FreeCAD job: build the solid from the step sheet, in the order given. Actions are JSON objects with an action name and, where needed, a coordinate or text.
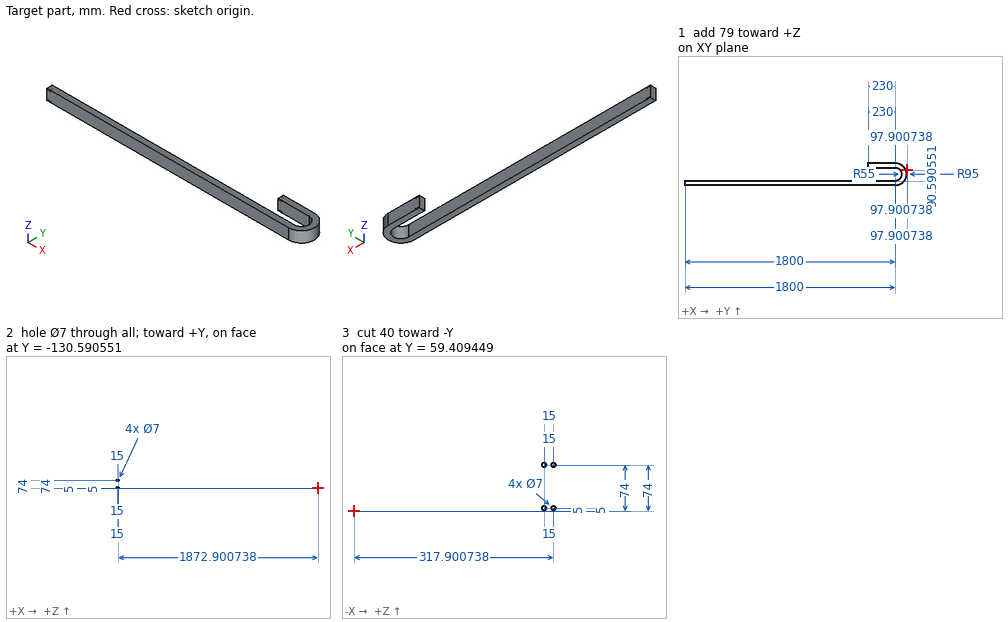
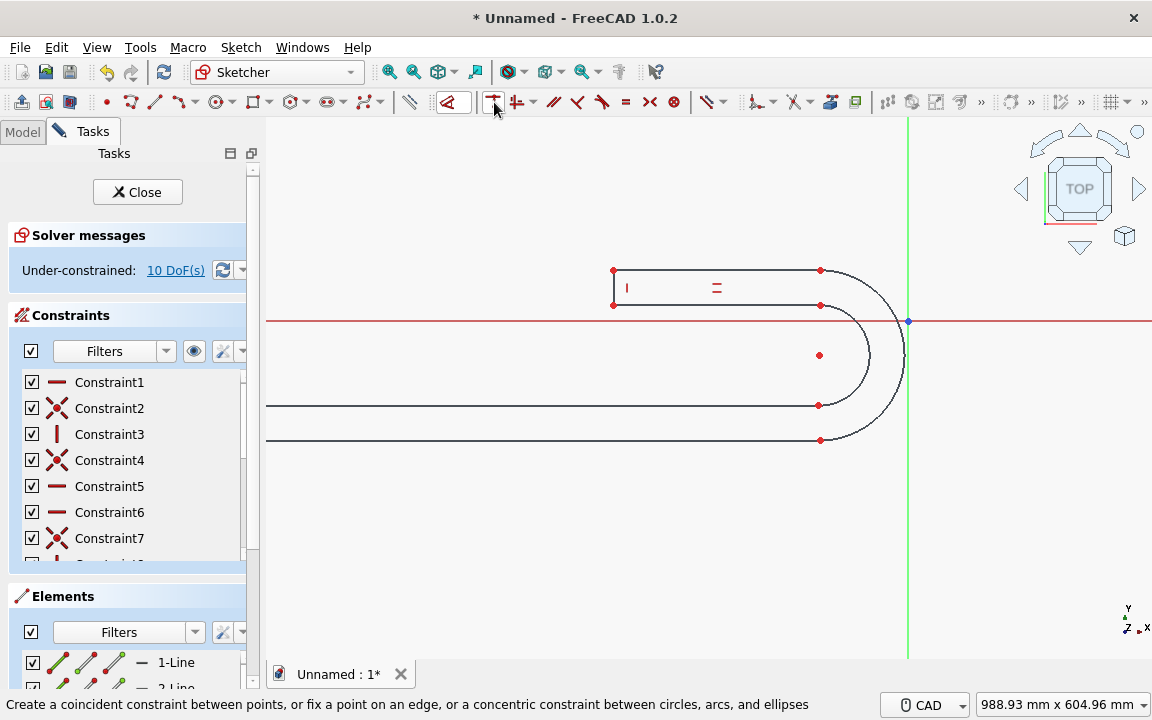
{"action": "key", "text": "d"}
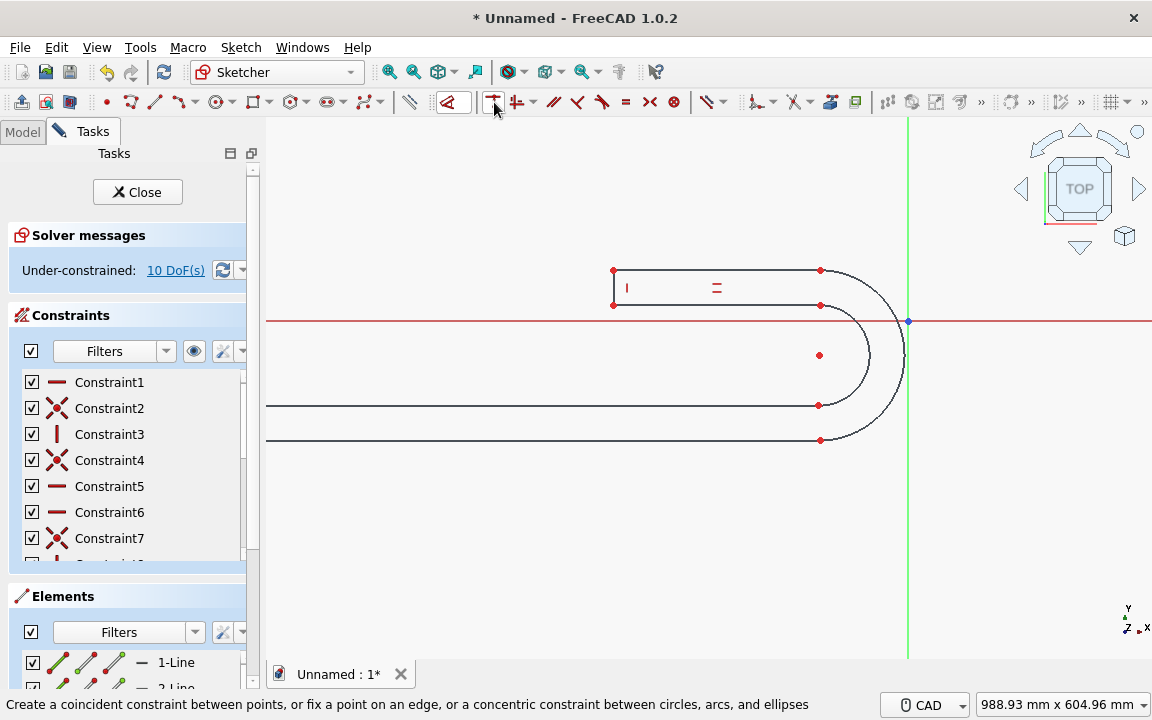
{"action": "left_click", "coordinate": [889, 405]}
{"action": "left_click", "coordinate": [871, 461]}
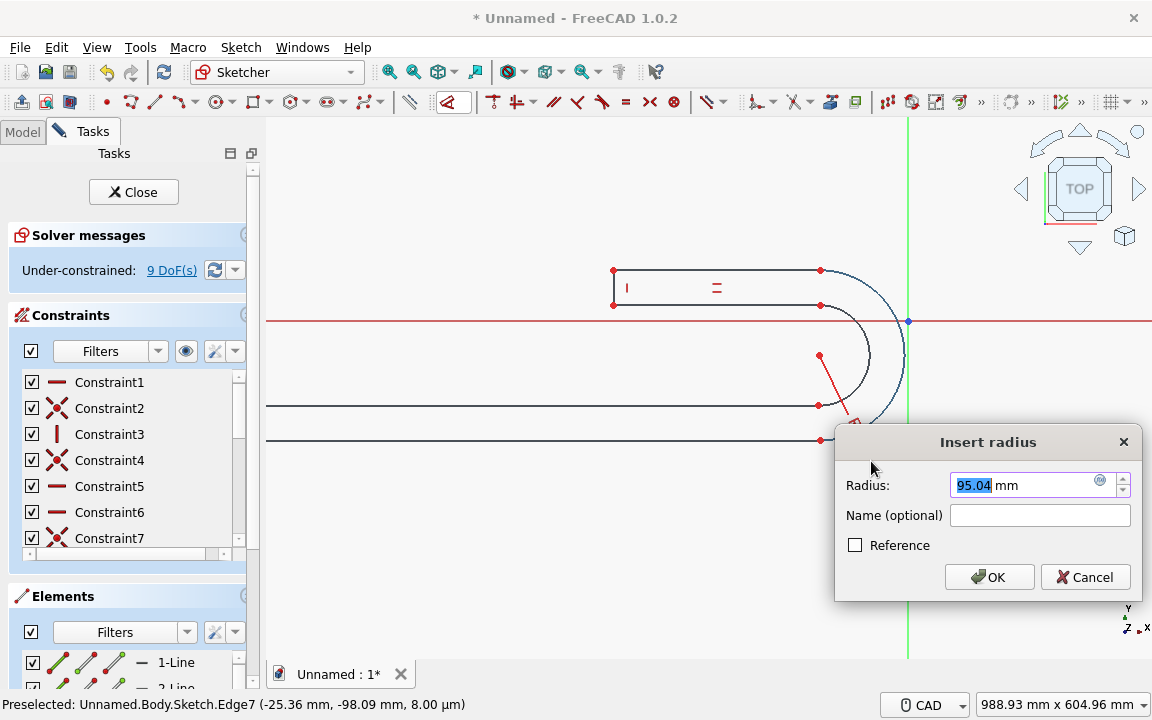
{"action": "type", "text": "95"}
{"action": "key", "text": "Return"}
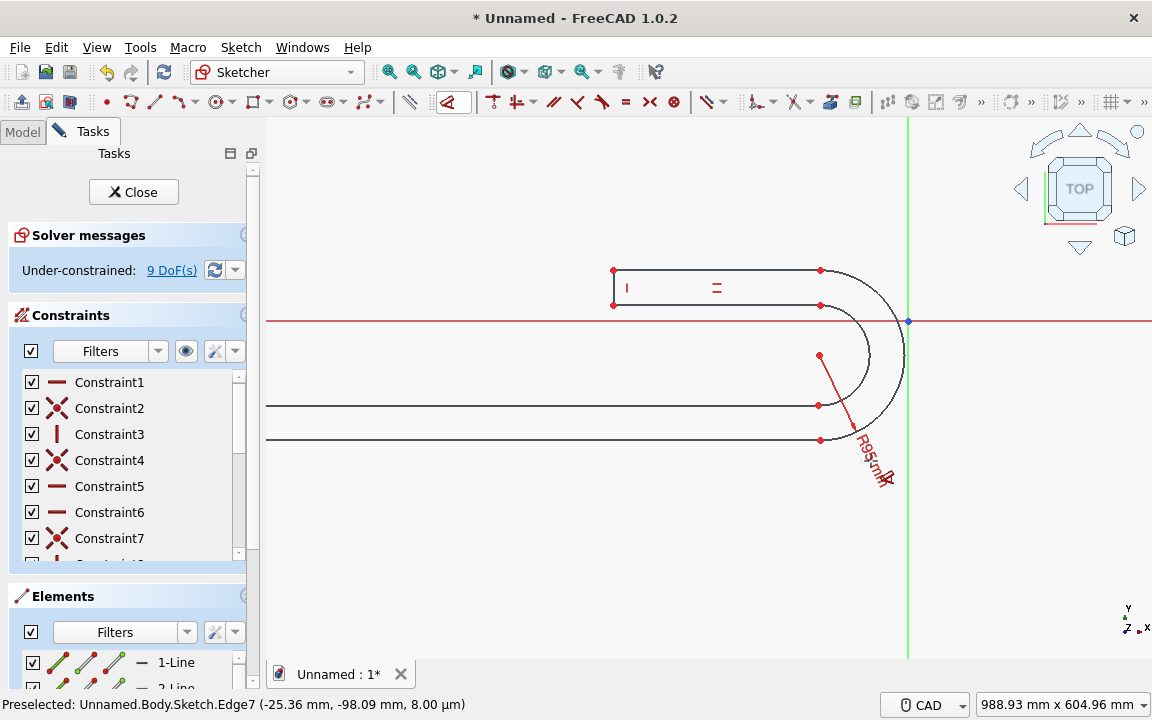
{"action": "left_click", "coordinate": [860, 385]}
{"action": "left_click", "coordinate": [771, 422]}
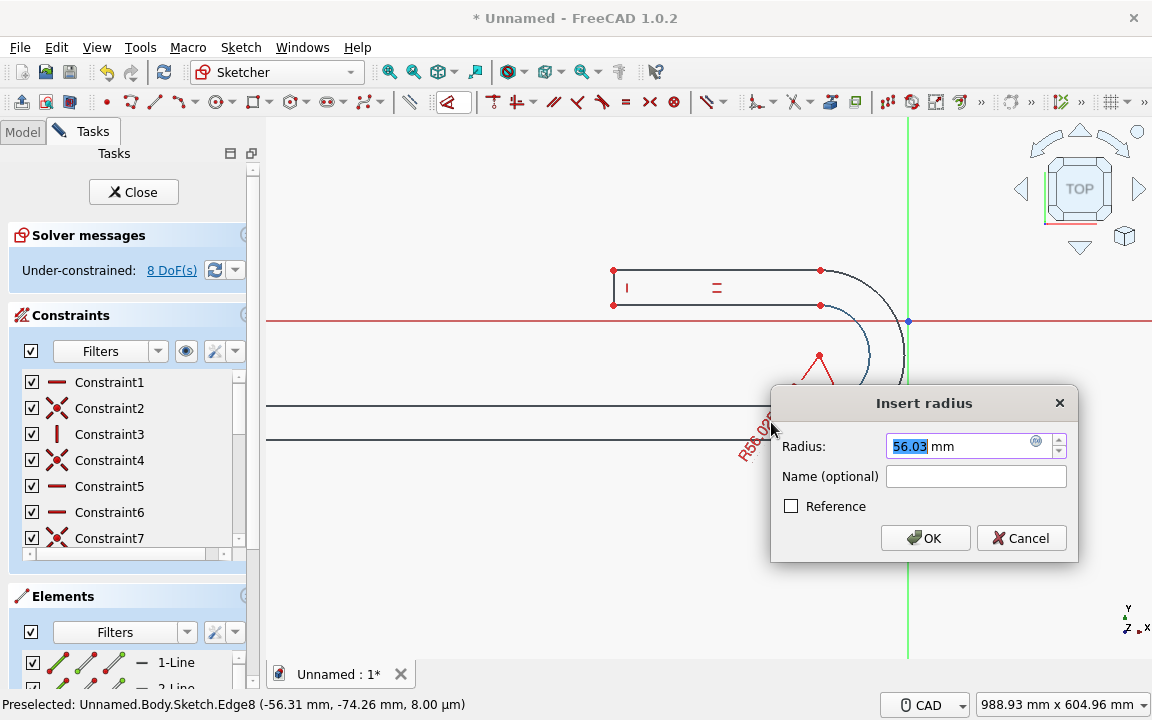
{"action": "type", "text": "55"}
{"action": "key", "text": "Return"}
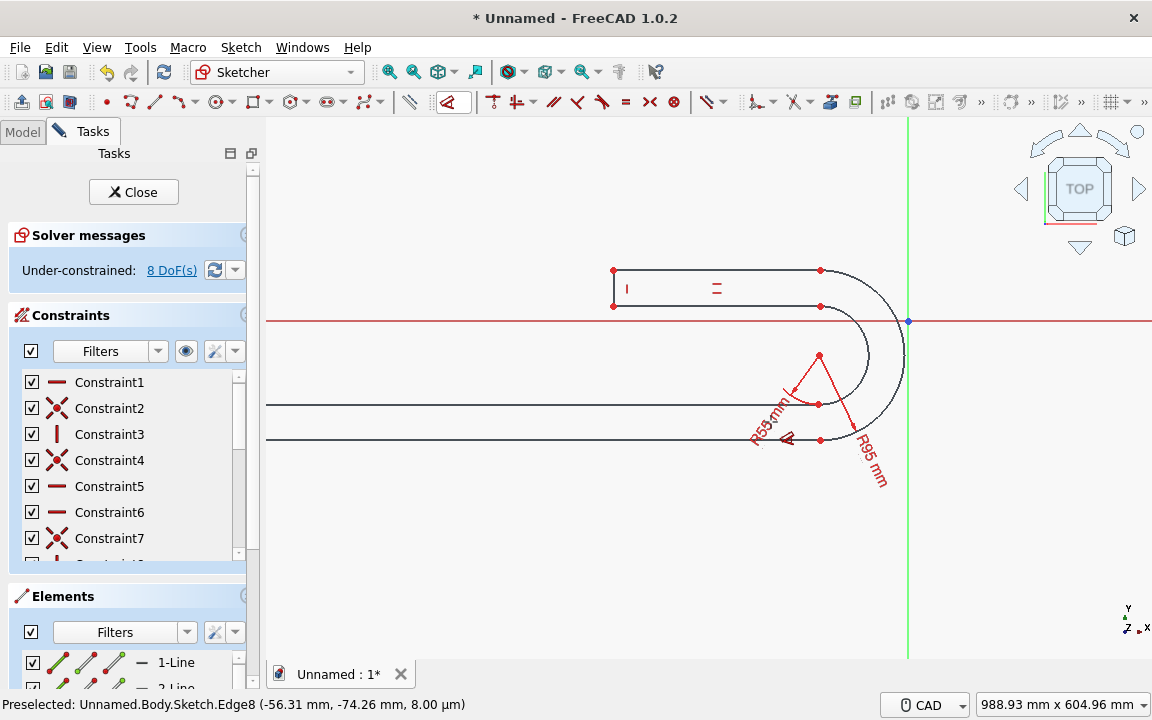
{"action": "left_click", "coordinate": [759, 270]}
{"action": "left_click", "coordinate": [717, 236]}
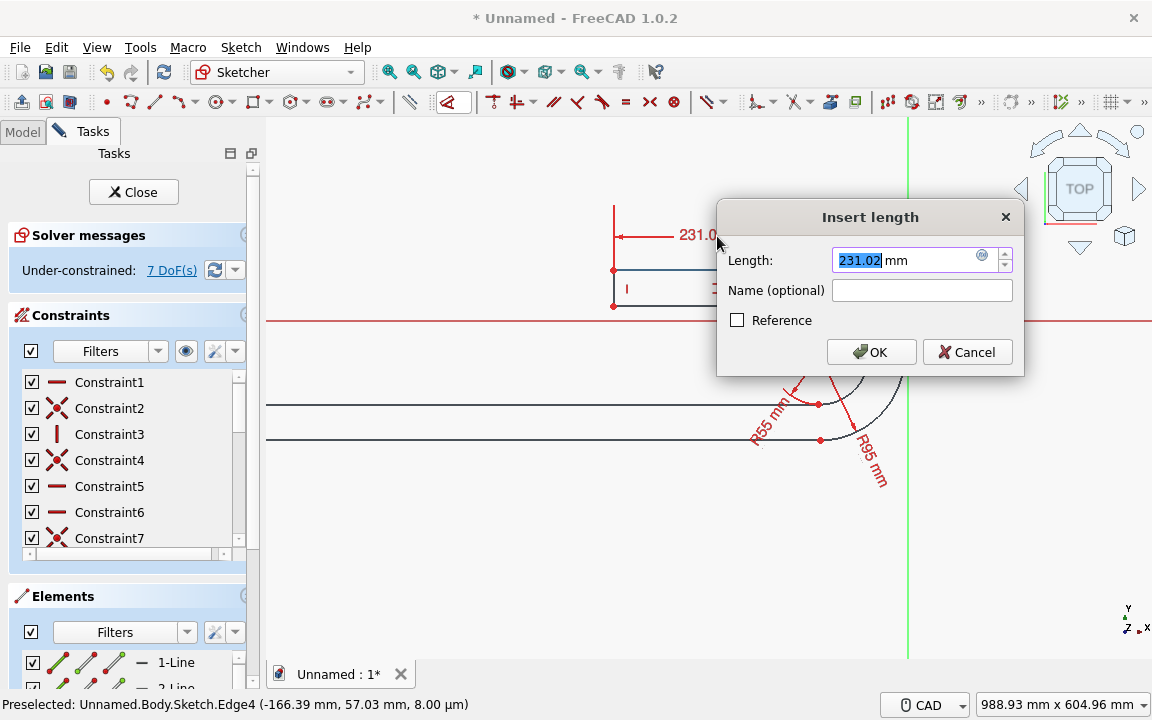
{"action": "type", "text": "230"}
{"action": "key", "text": "Return"}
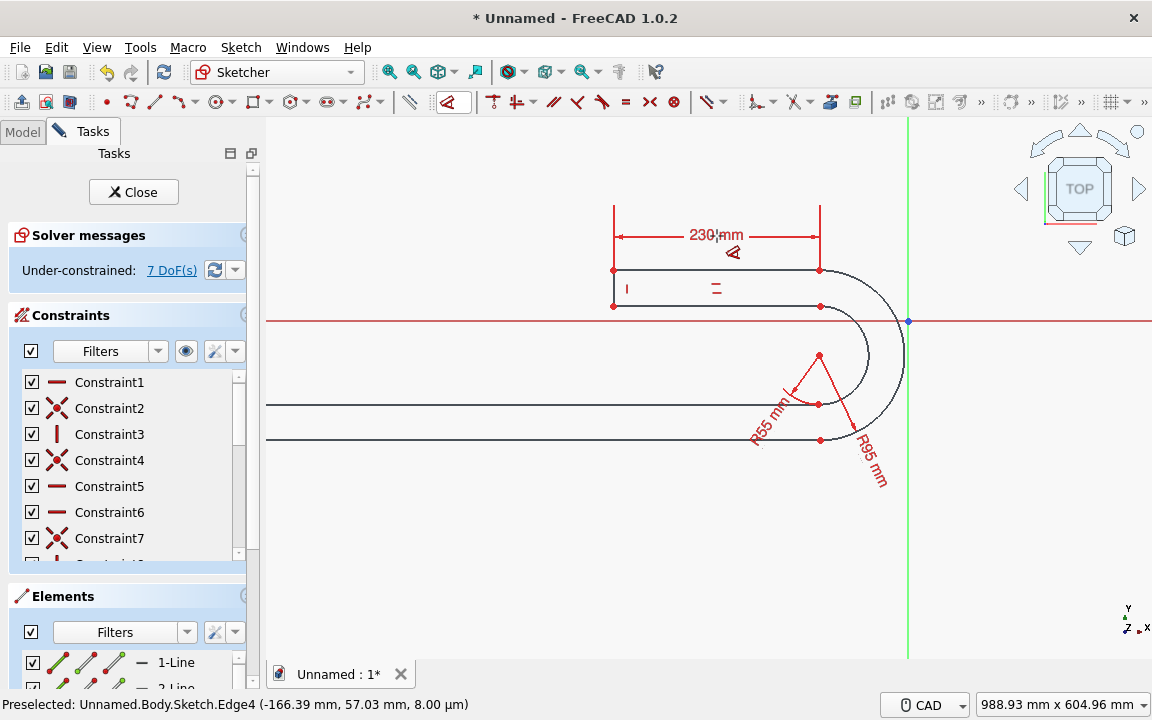
{"action": "left_click", "coordinate": [676, 306]}
{"action": "left_click", "coordinate": [717, 340]}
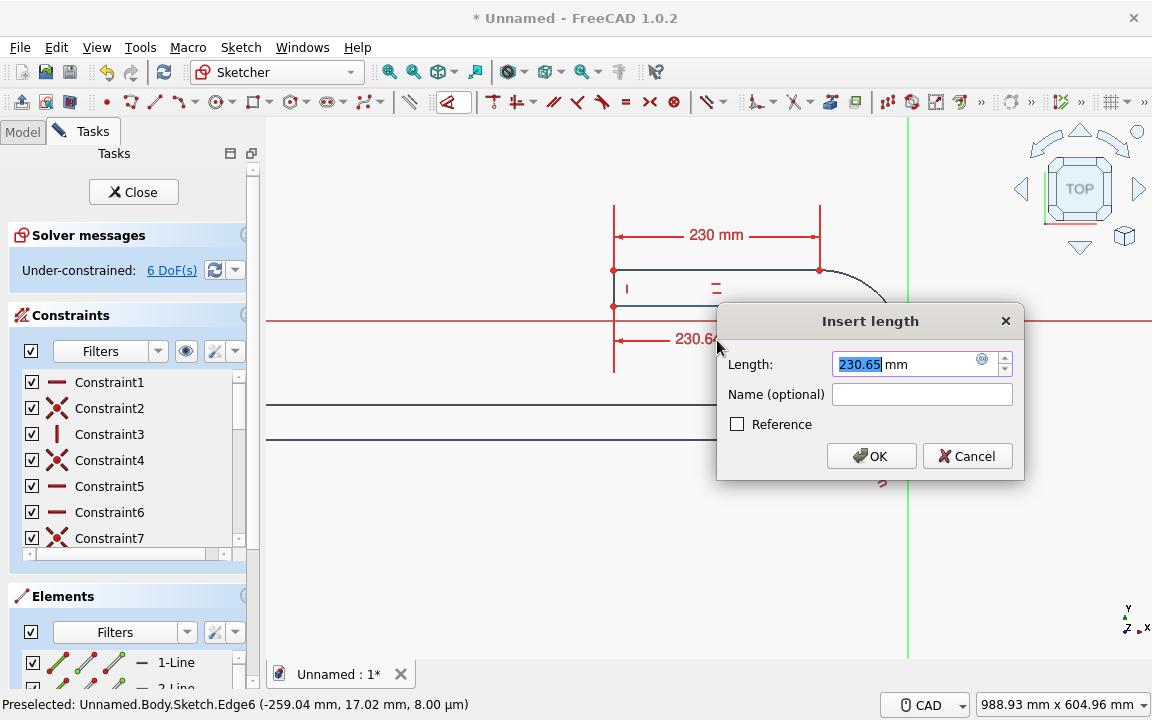
{"action": "type", "text": "230"}
{"action": "key", "text": "Return"}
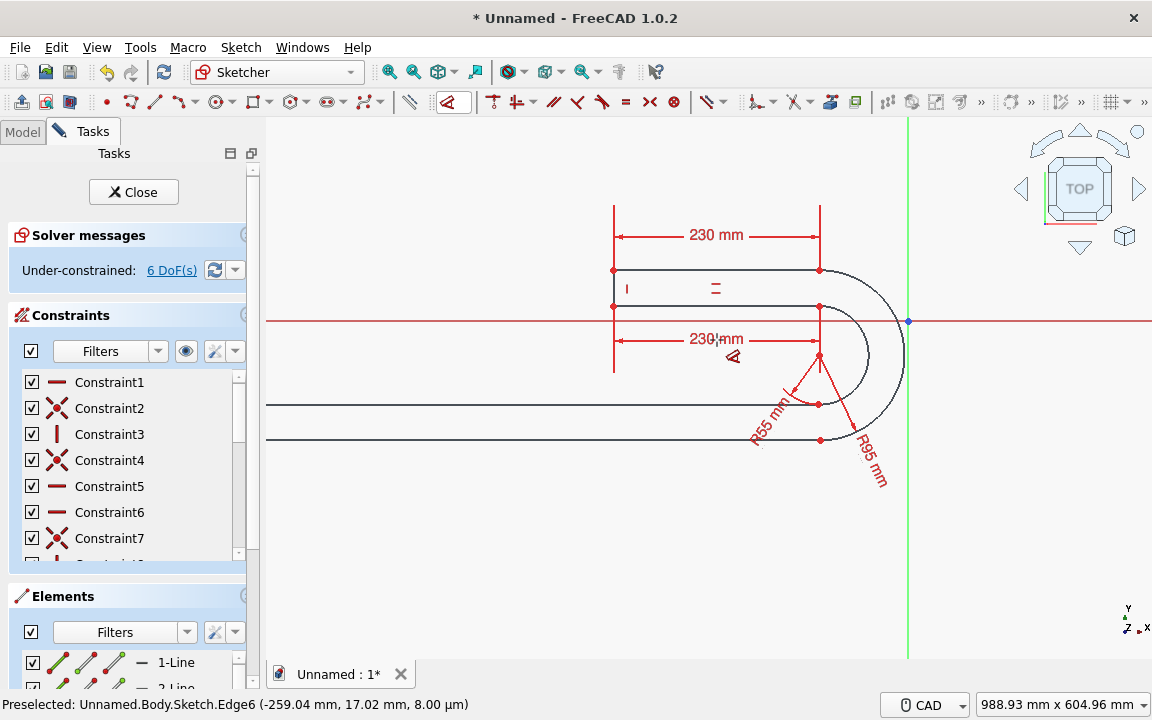
{"action": "left_click", "coordinate": [336, 405]}
{"action": "left_click", "coordinate": [556, 371]}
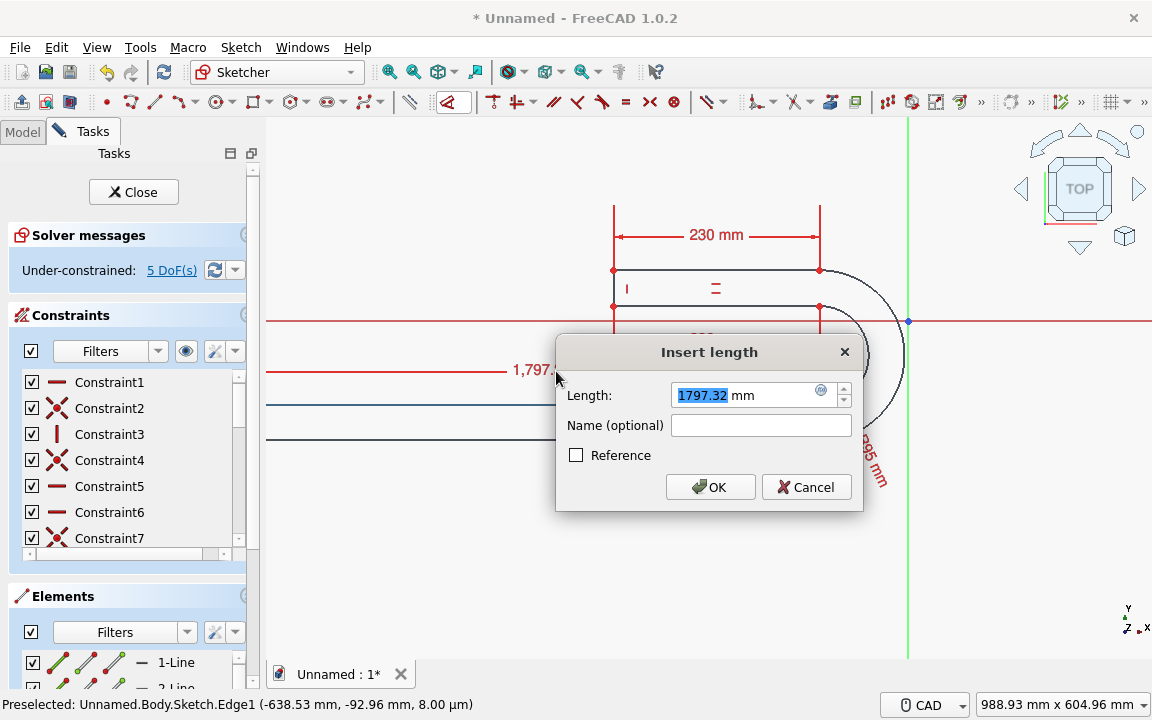
{"action": "type", "text": "1800"}
{"action": "key", "text": "Return"}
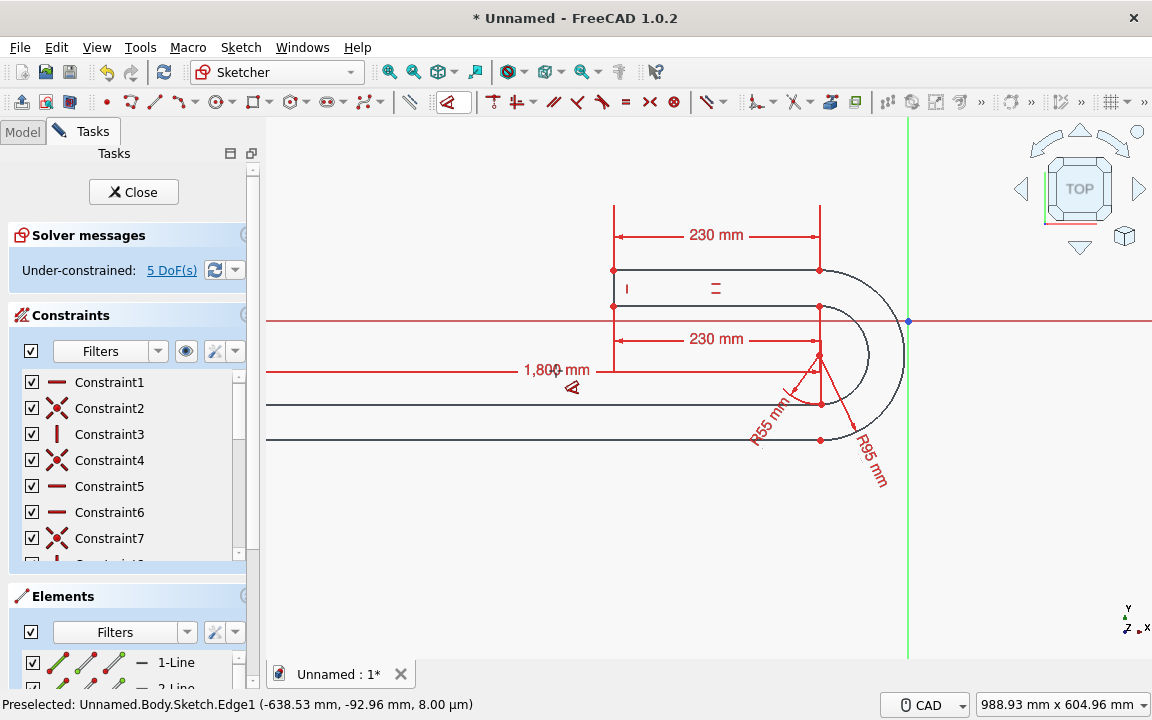
{"action": "left_click", "coordinate": [337, 440]}
{"action": "left_click", "coordinate": [557, 474]}